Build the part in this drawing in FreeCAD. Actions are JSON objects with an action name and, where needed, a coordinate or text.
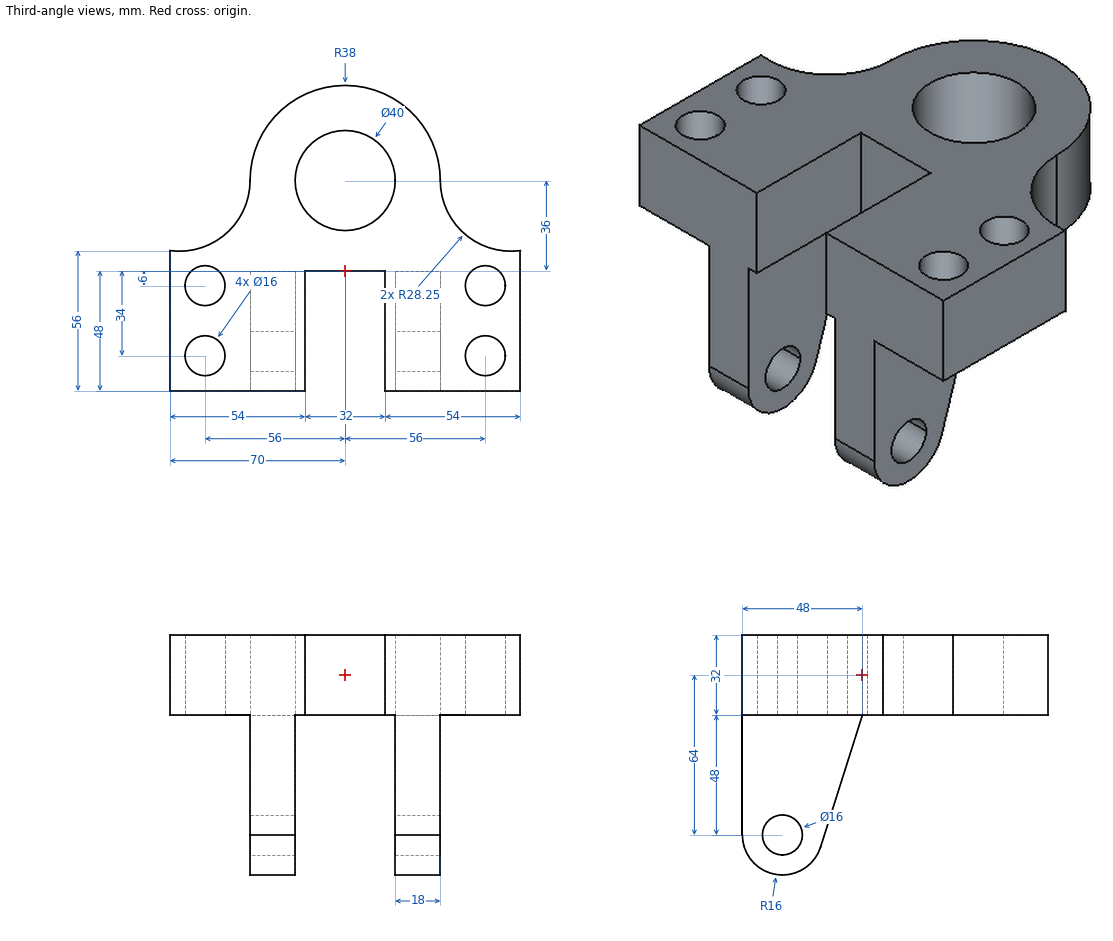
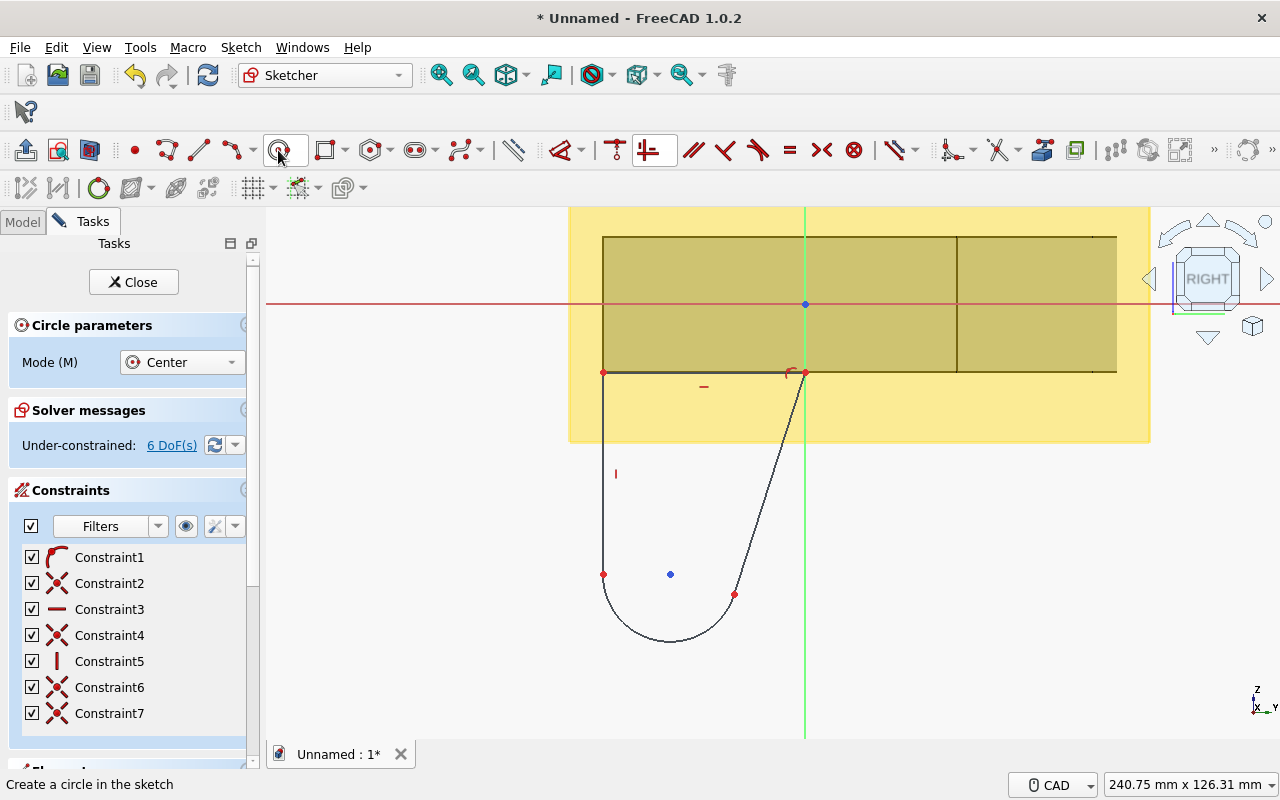
{"action": "left_click", "coordinate": [670, 574]}
{"action": "mouse_move", "coordinate": [694, 550]}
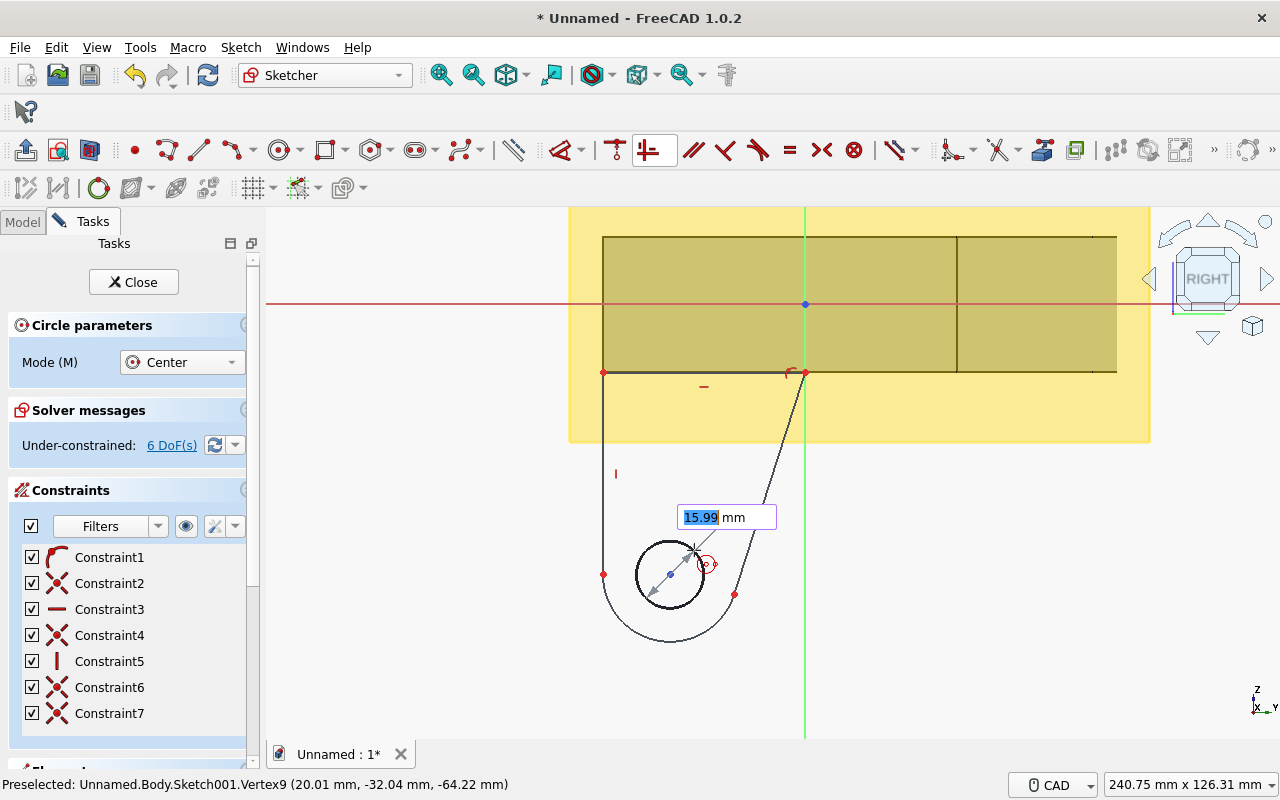
{"action": "type", "text": "16"}
{"action": "key", "text": "Return"}
{"action": "key", "text": "Escape"}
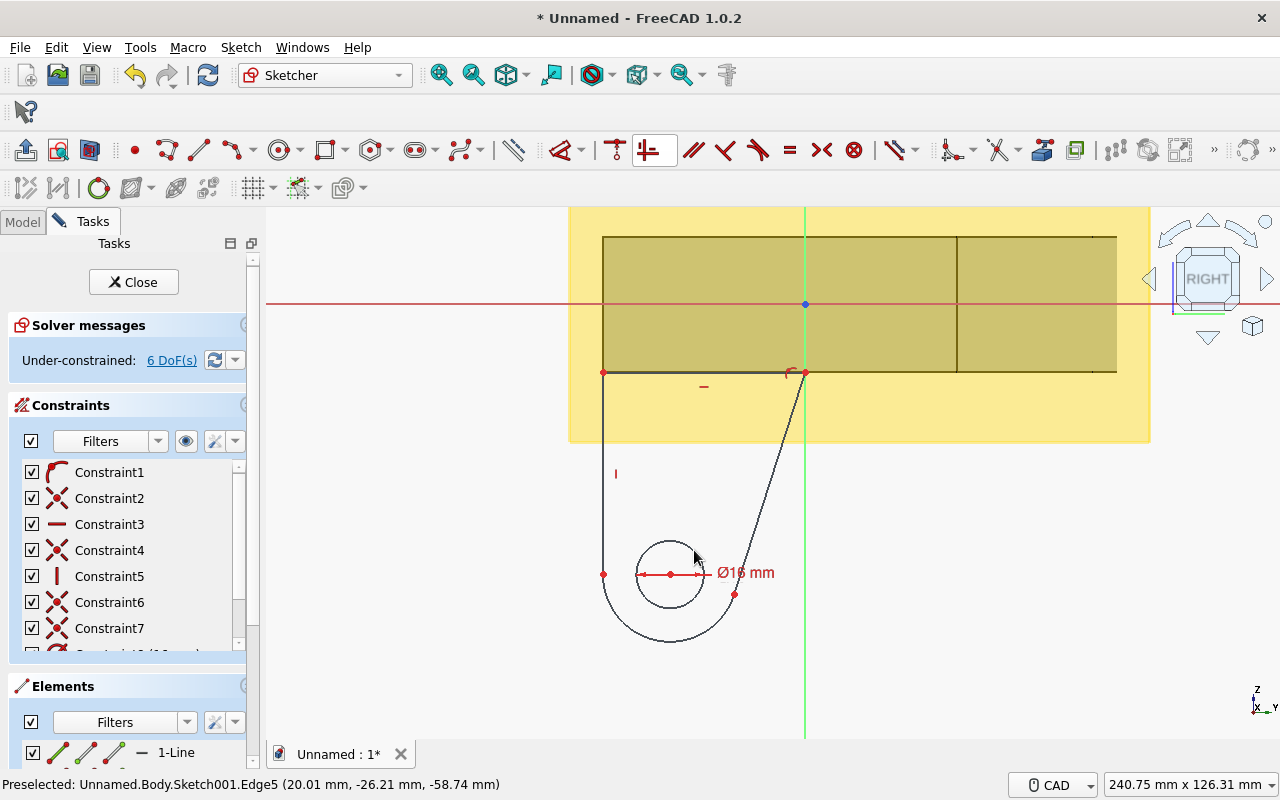
{"action": "left_click", "coordinate": [755, 528]}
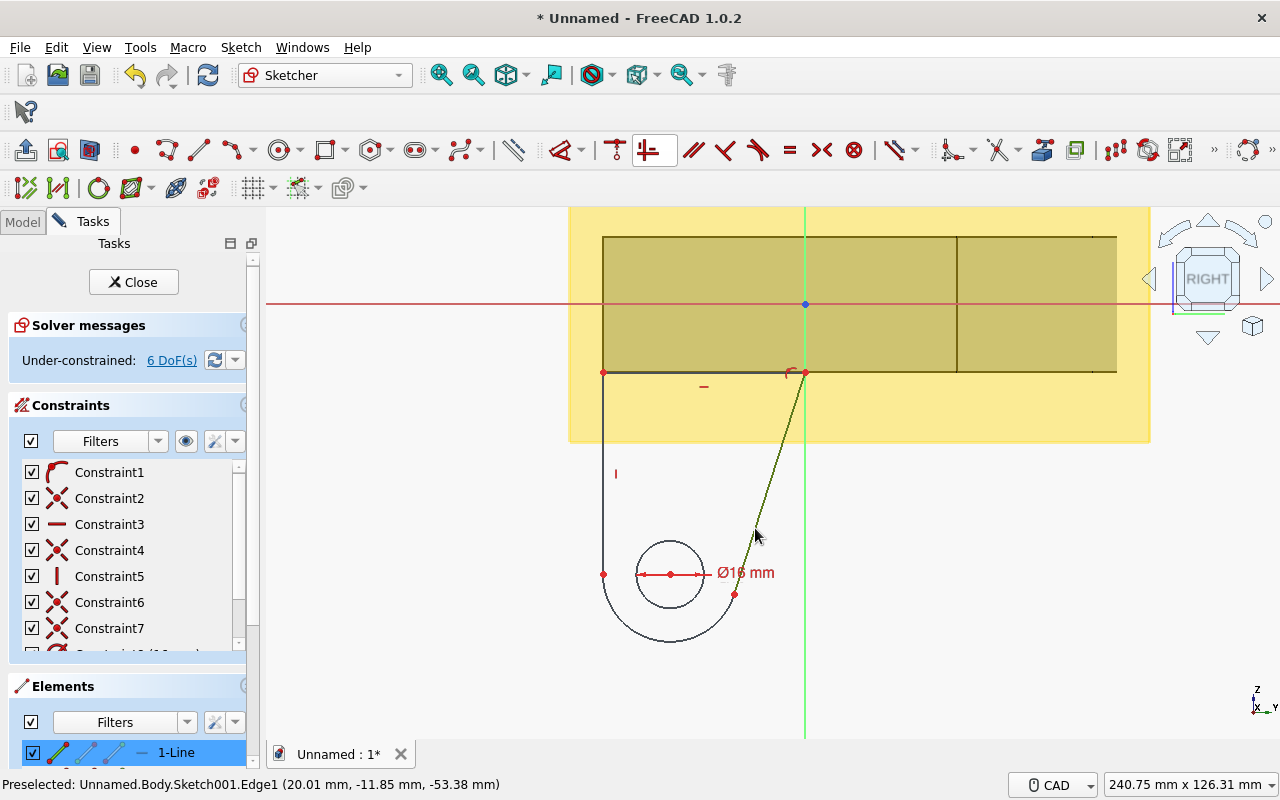
{"action": "left_click", "coordinate": [626, 625]}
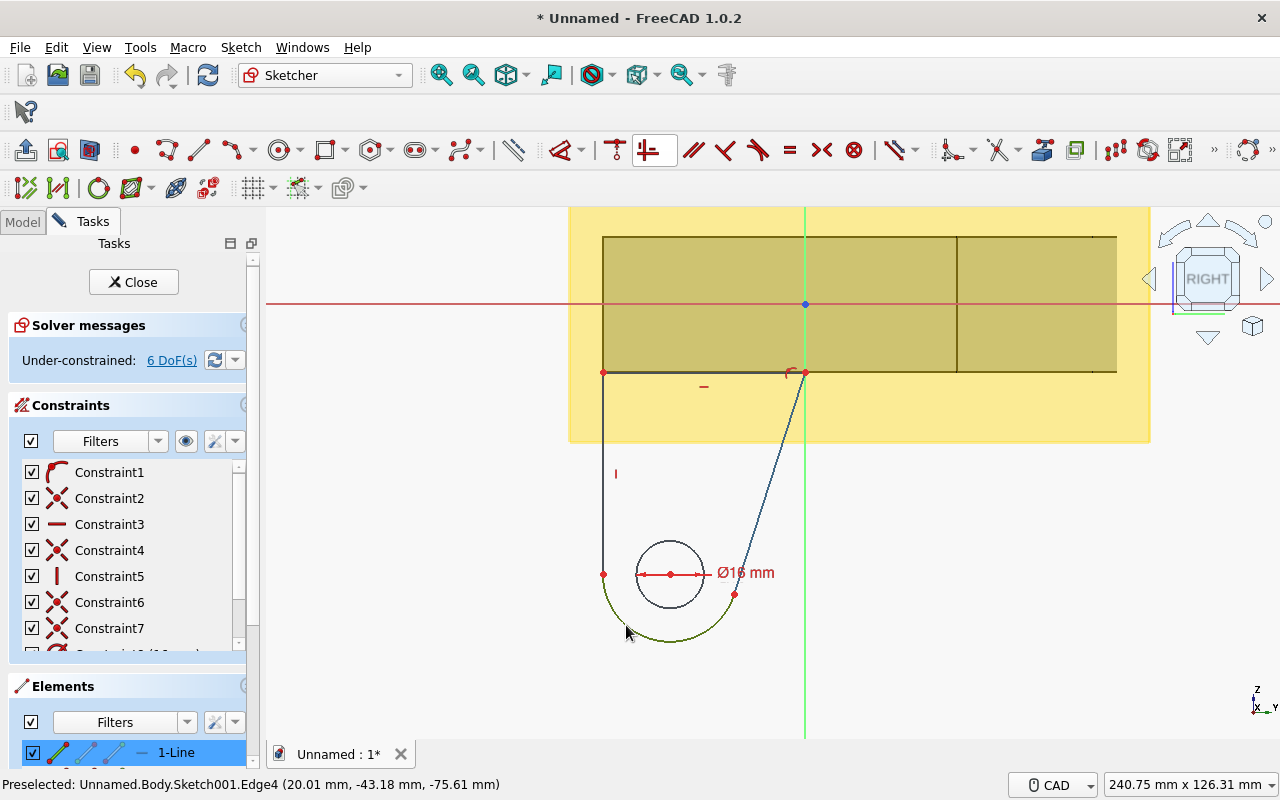
{"action": "left_click", "coordinate": [758, 150]}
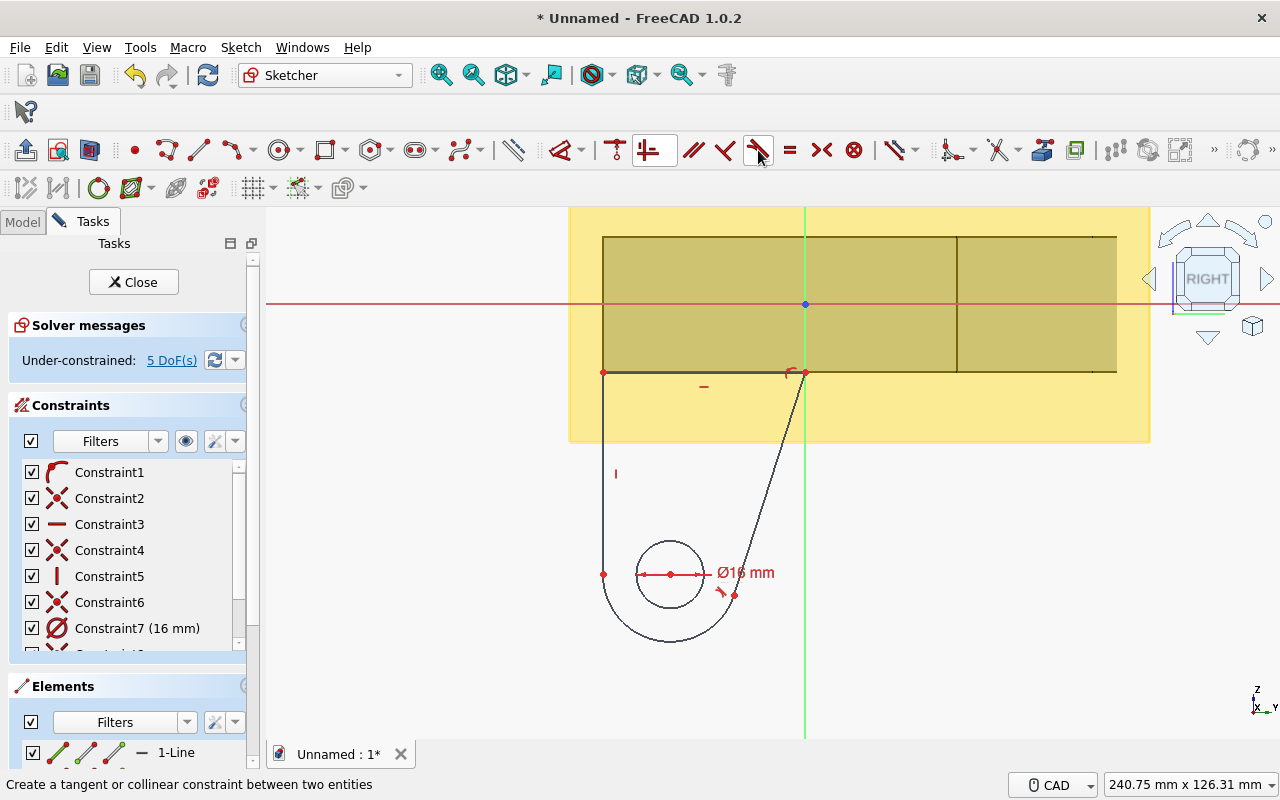
{"action": "left_click", "coordinate": [603, 434]}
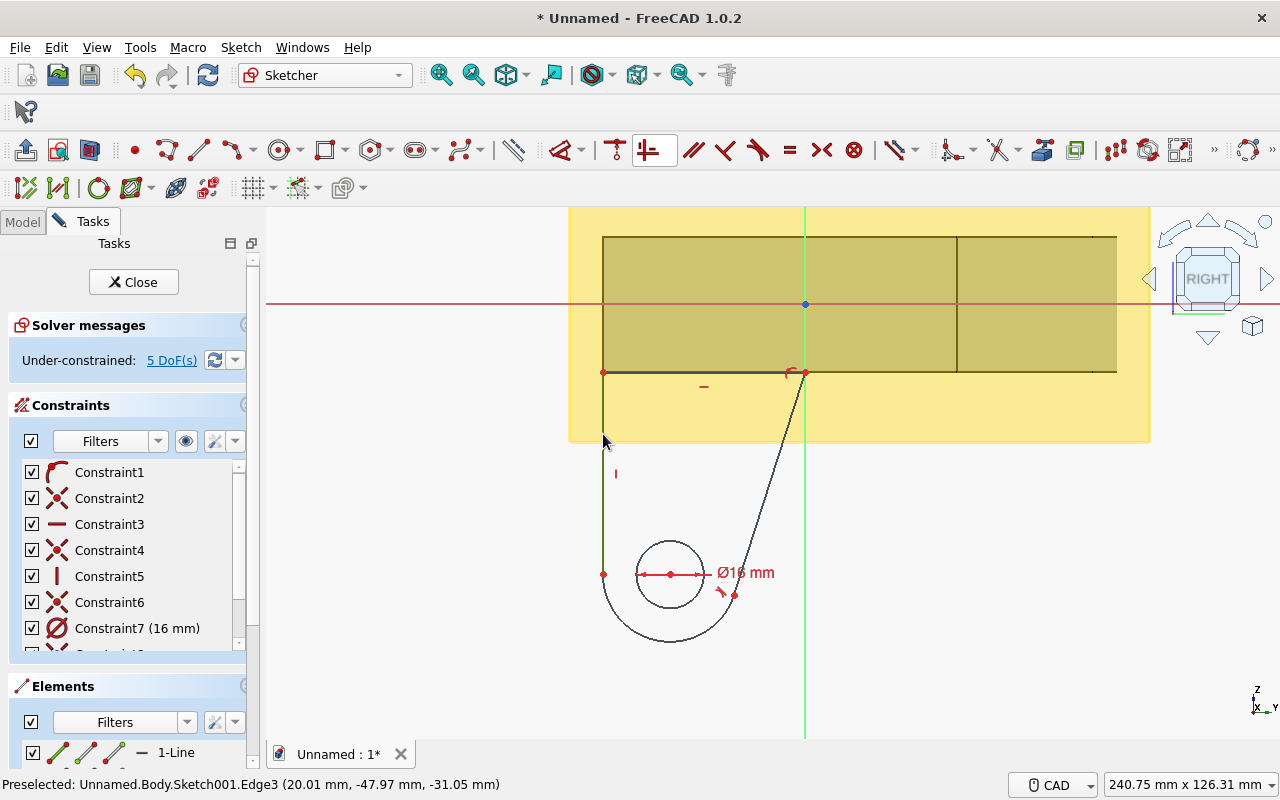
{"action": "left_click", "coordinate": [626, 625]}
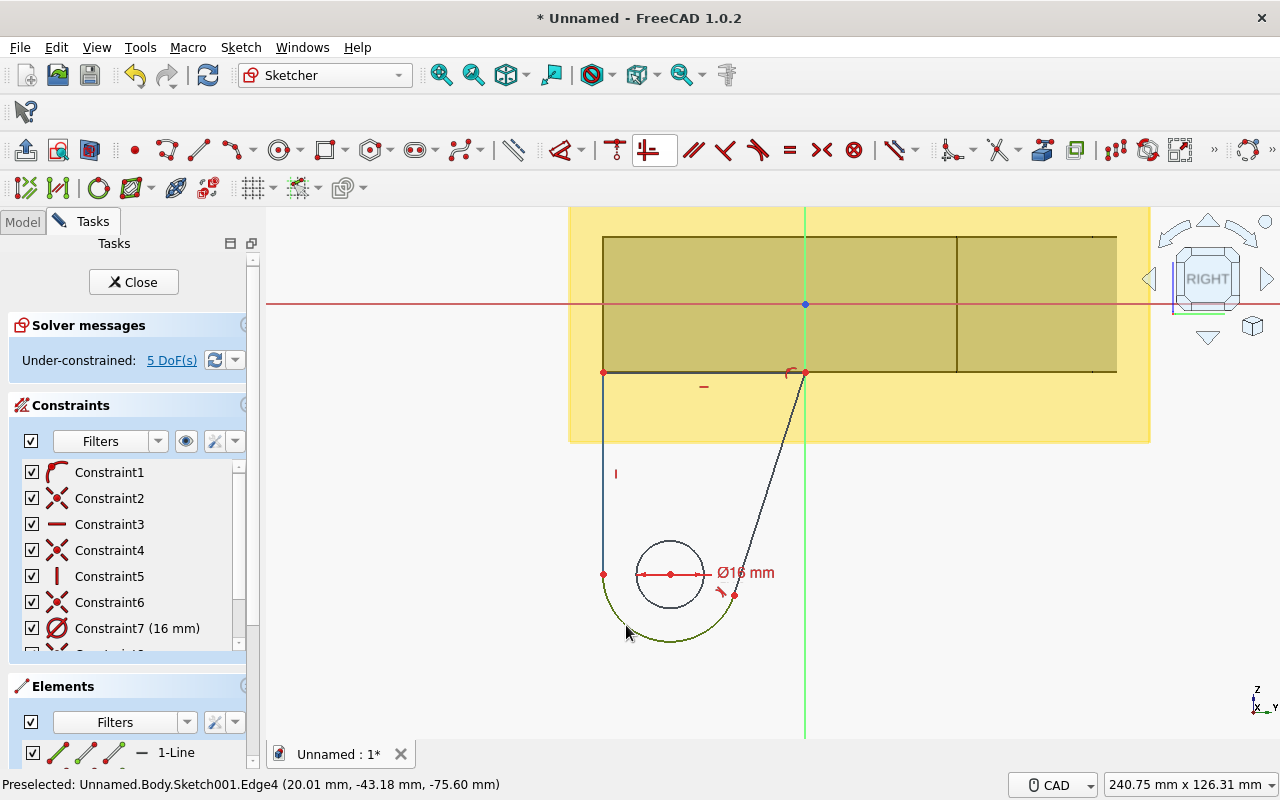
{"action": "left_click", "coordinate": [758, 150]}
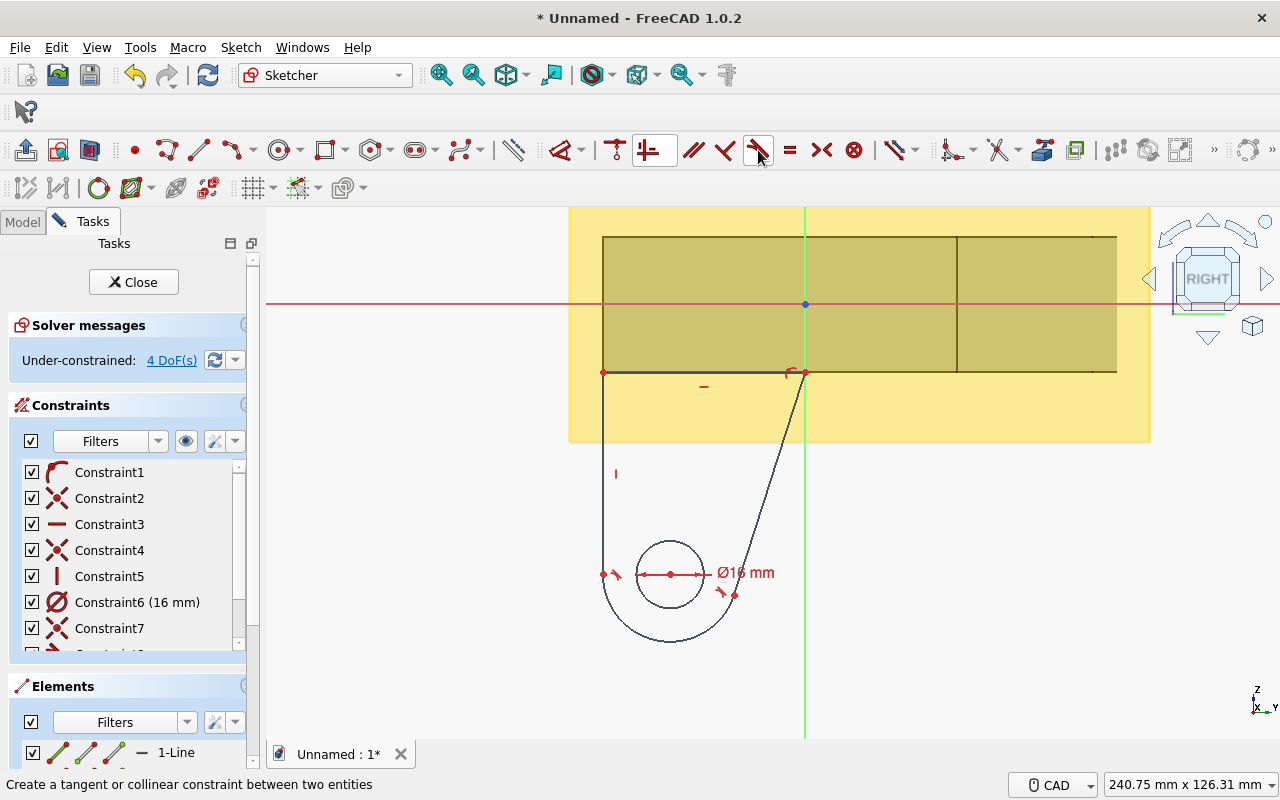
{"action": "left_click", "coordinate": [560, 150]}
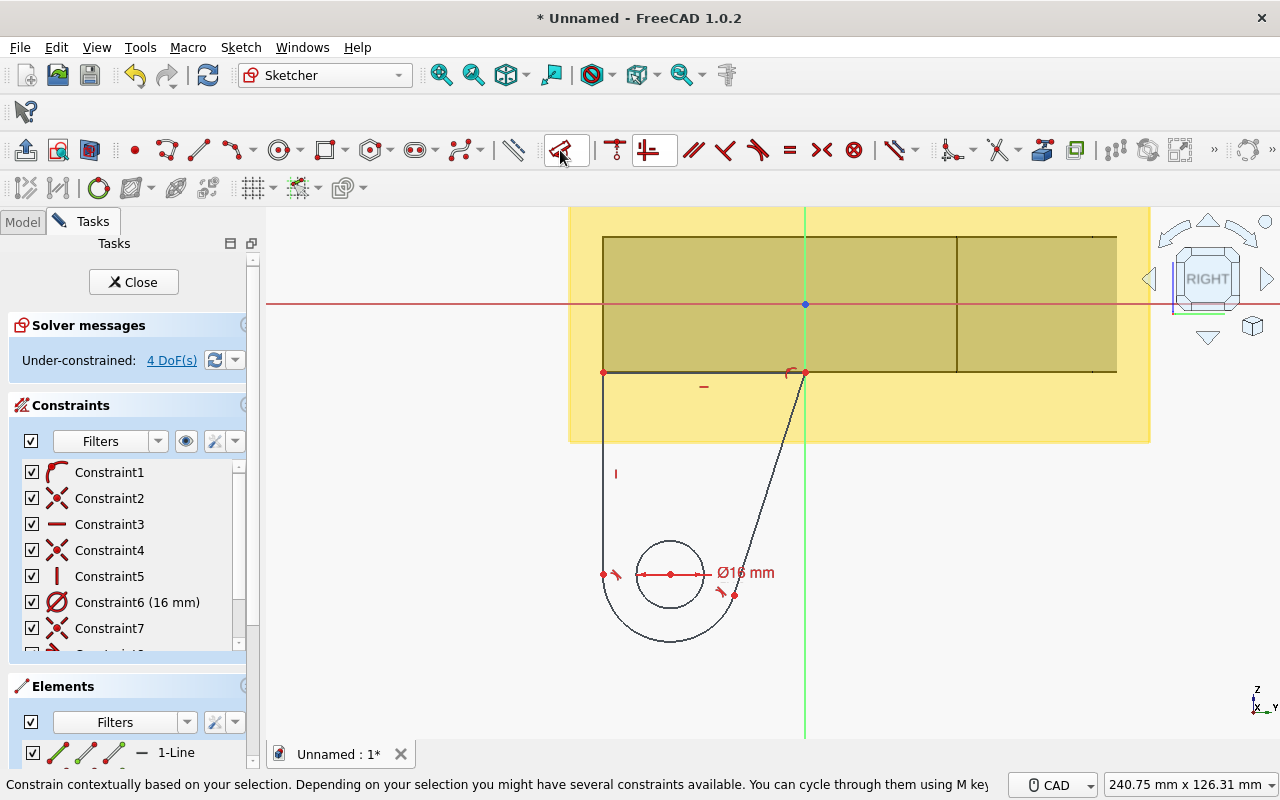
{"action": "left_click", "coordinate": [626, 625]}
{"action": "left_click", "coordinate": [605, 649]}